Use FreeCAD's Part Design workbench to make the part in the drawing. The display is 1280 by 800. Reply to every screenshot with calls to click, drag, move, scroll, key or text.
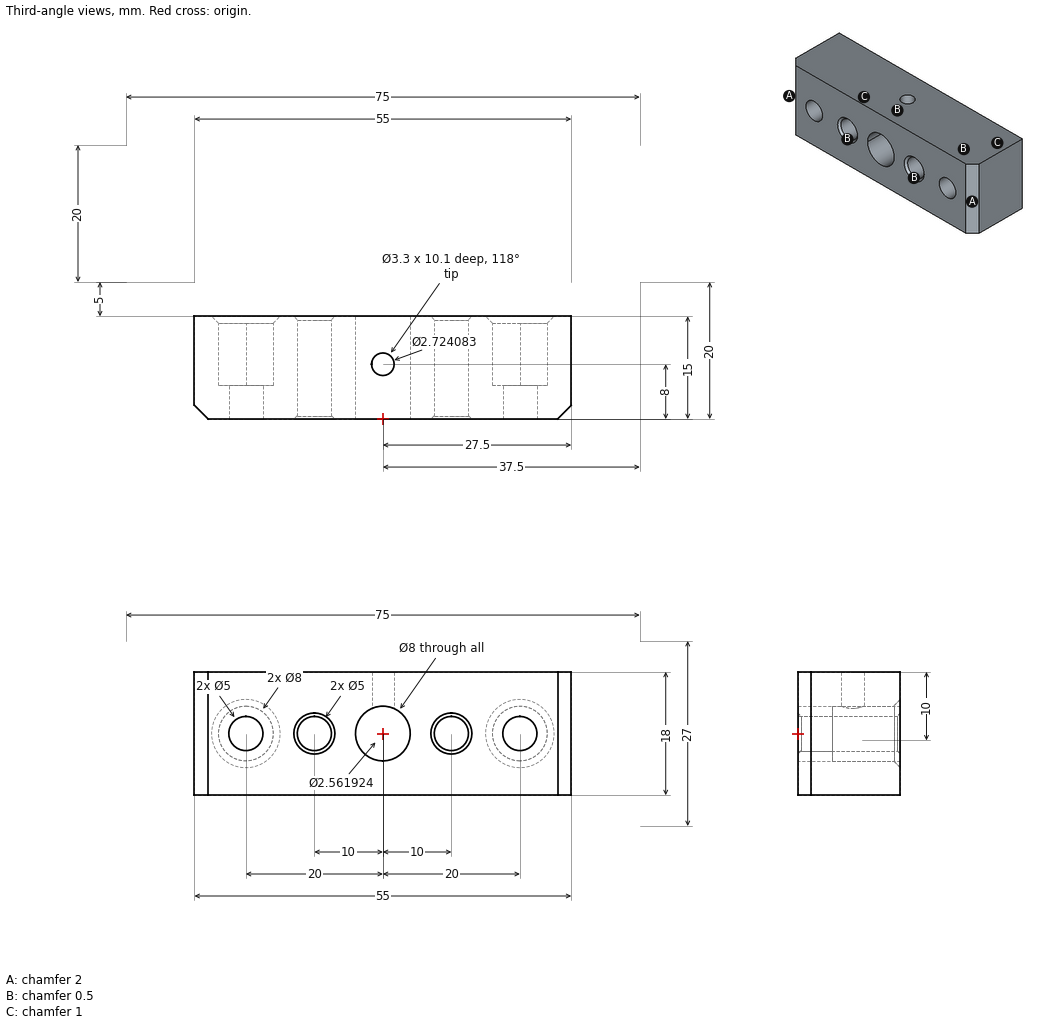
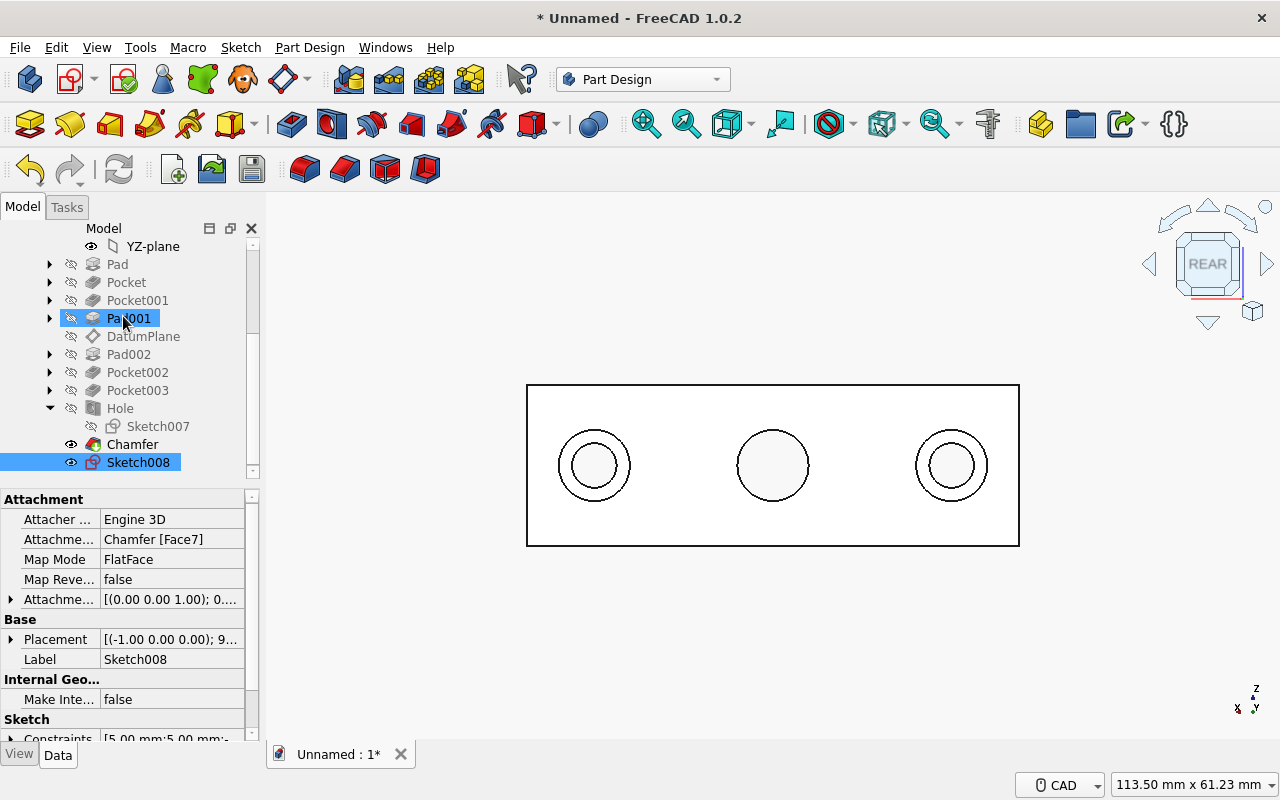
click(292, 124)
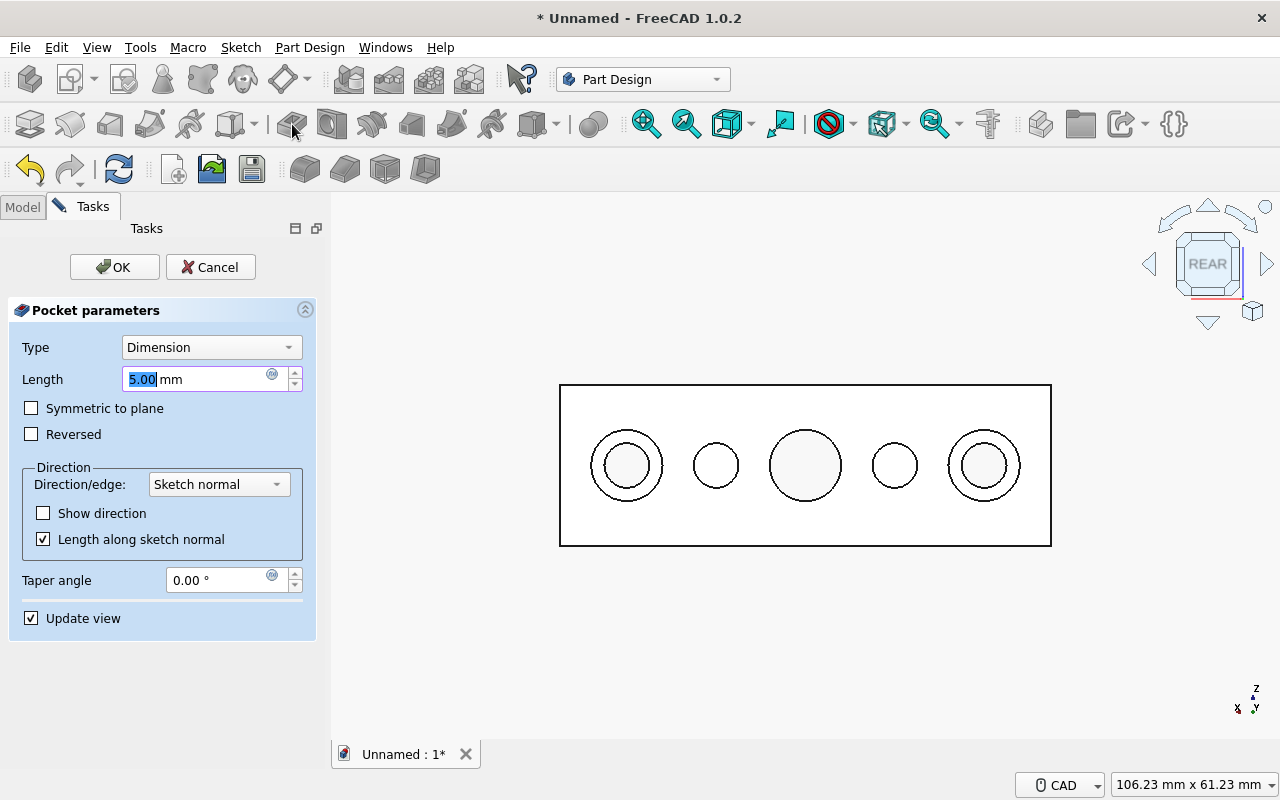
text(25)
key(Tab)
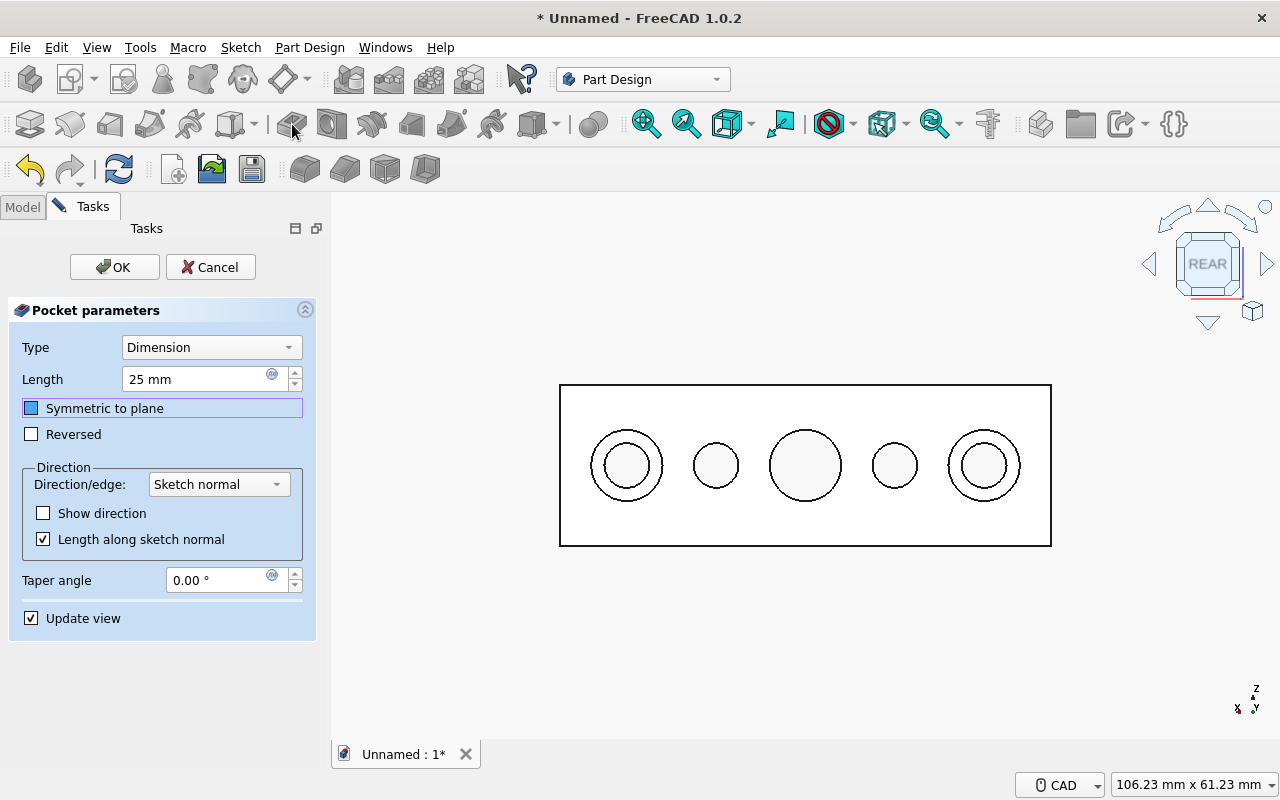
click(115, 267)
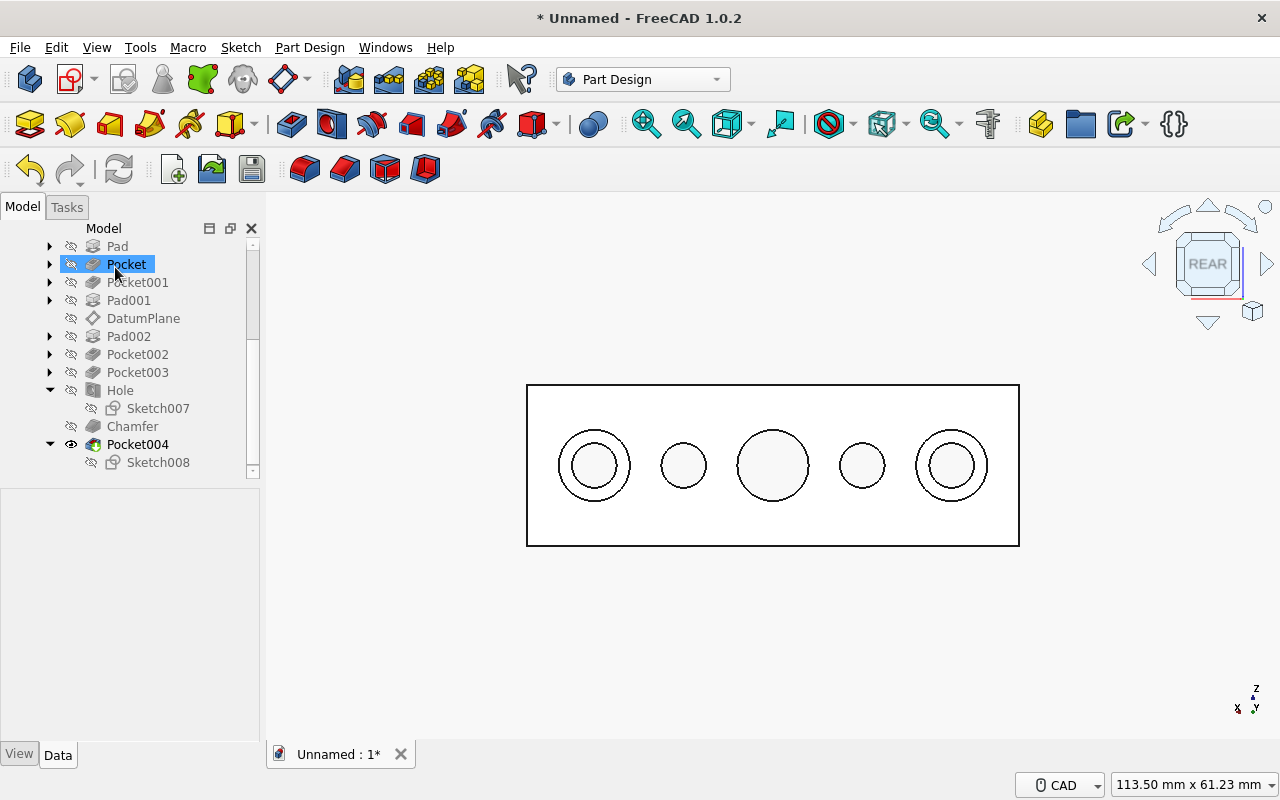
key(0)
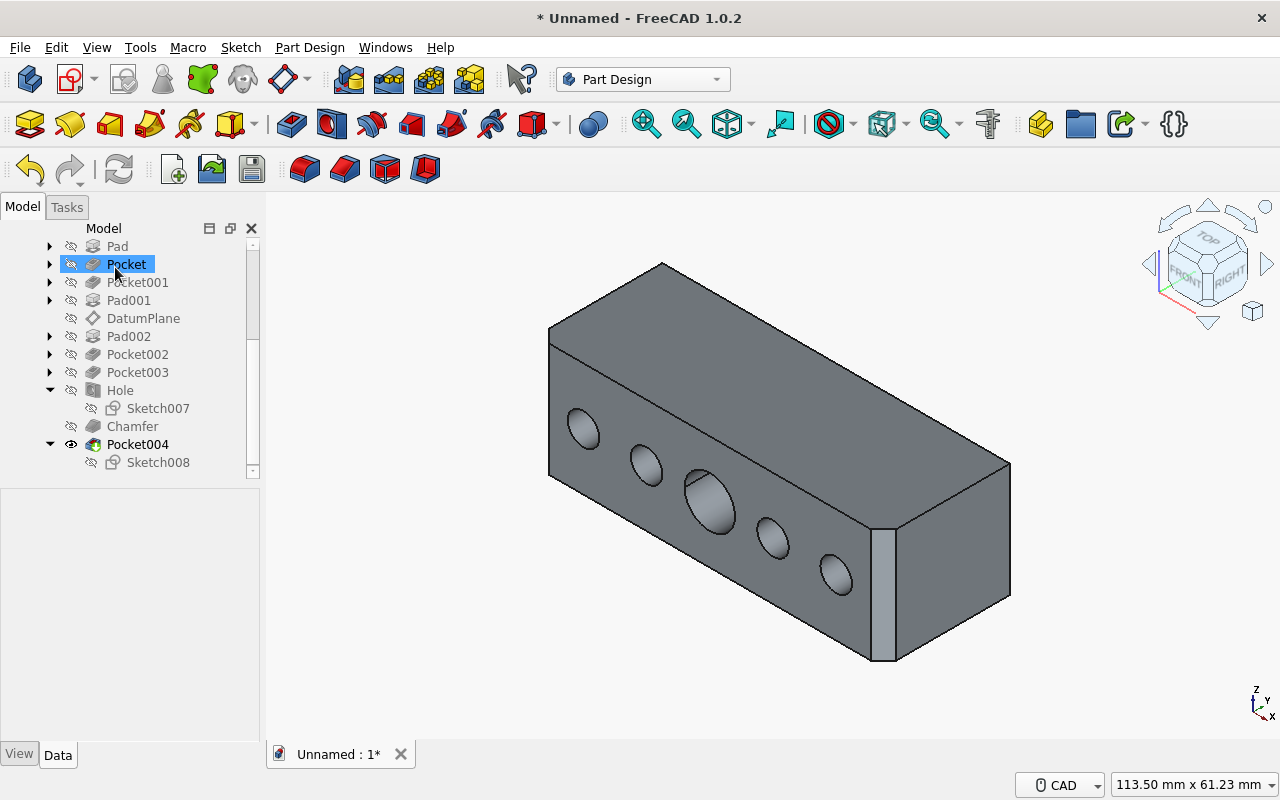
click(872, 456)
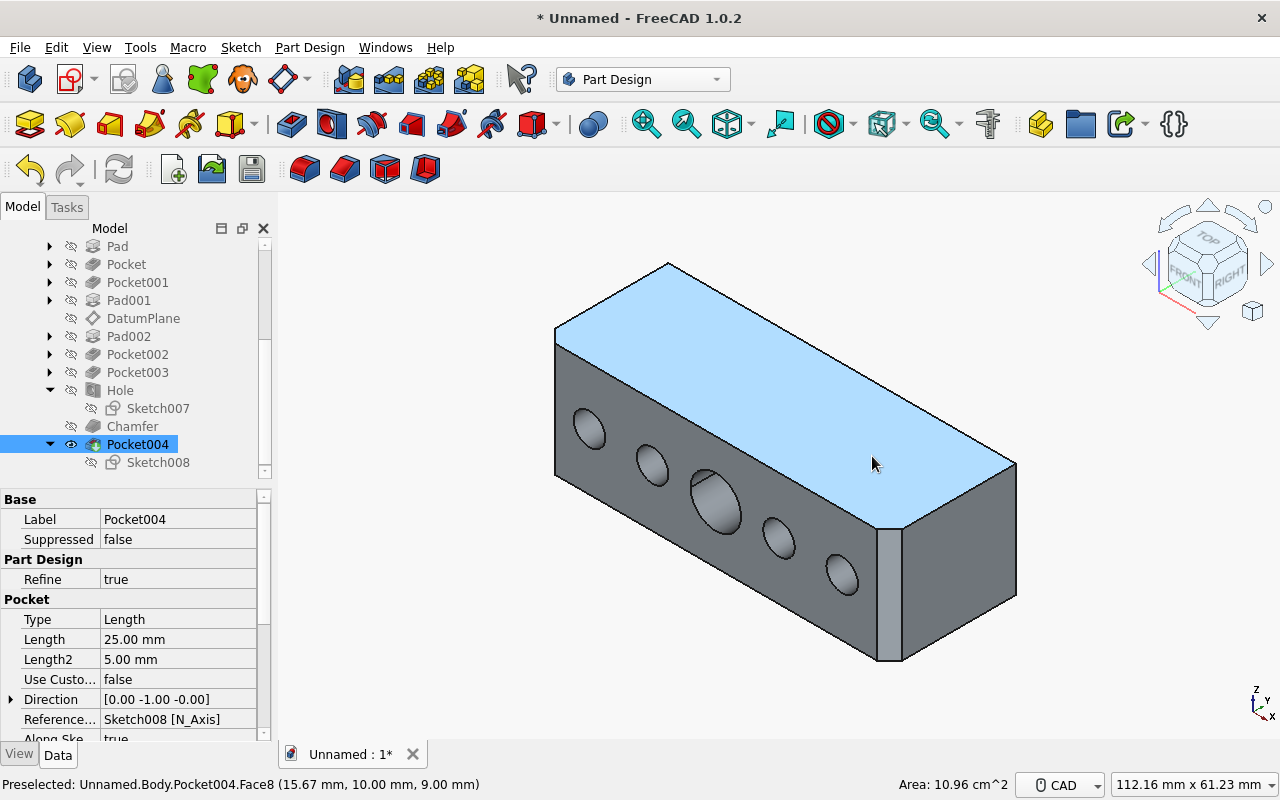
click(70, 80)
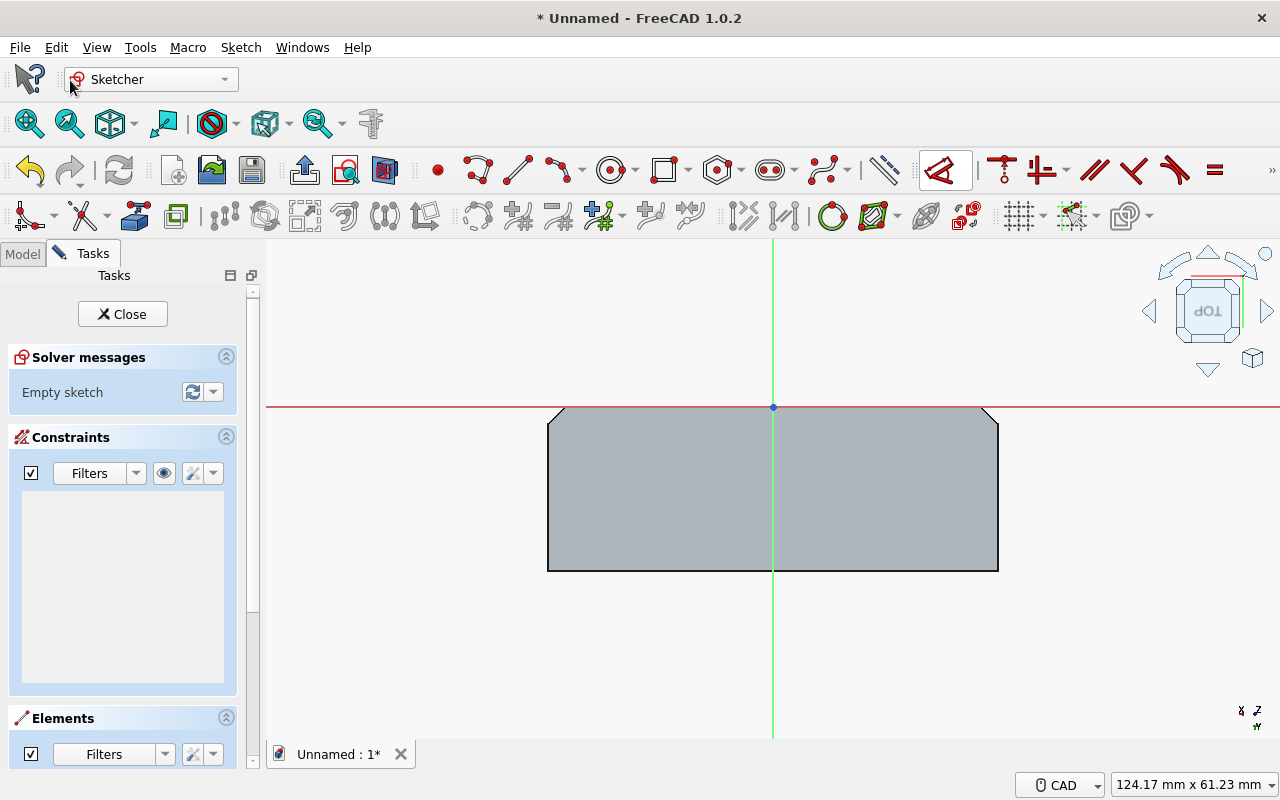
scroll(778, 471, up, 13)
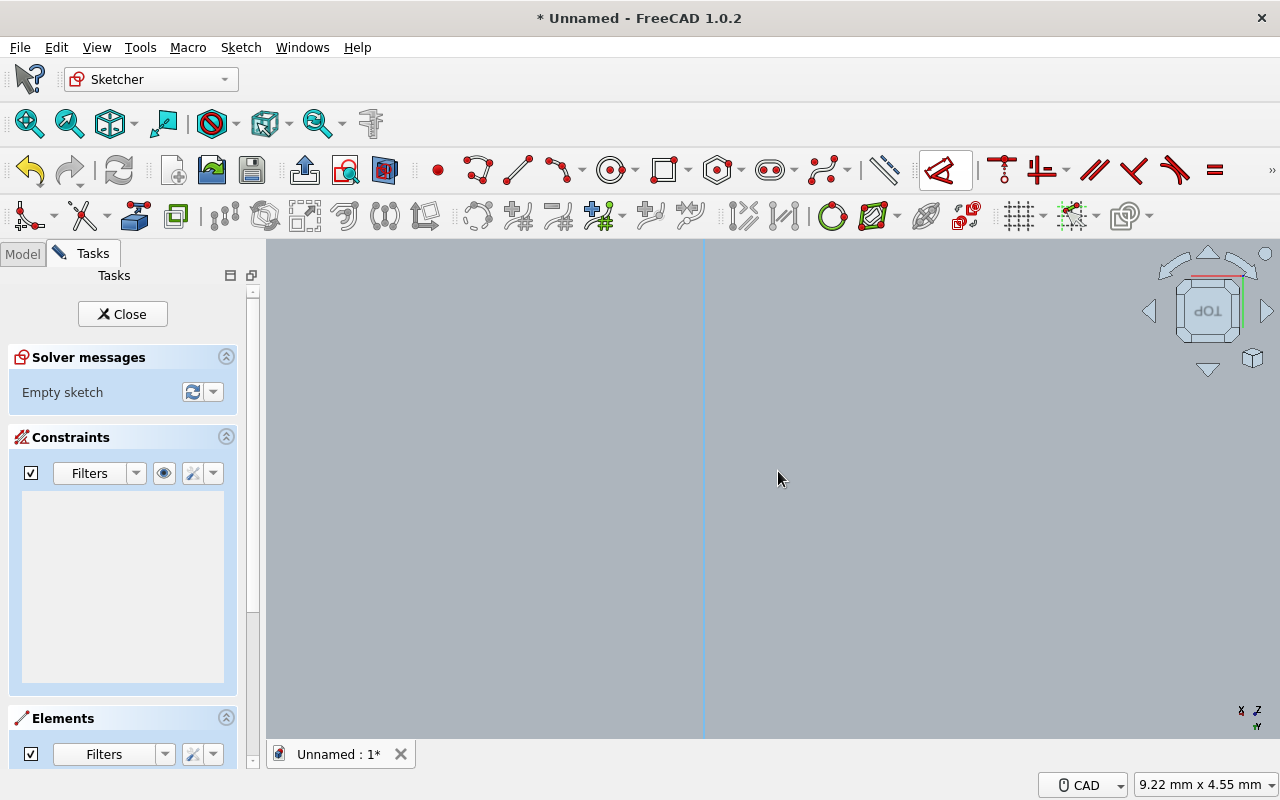
click(612, 170)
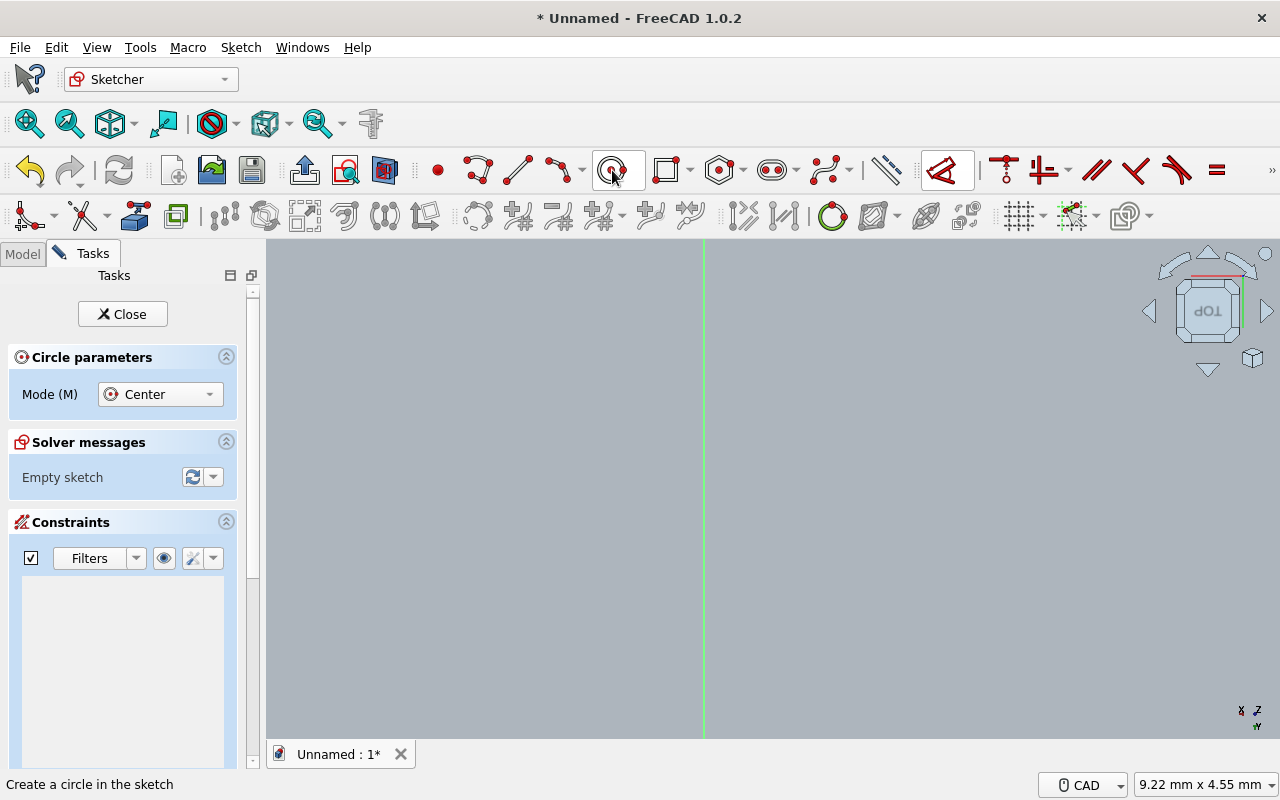
click(704, 488)
move(810, 382)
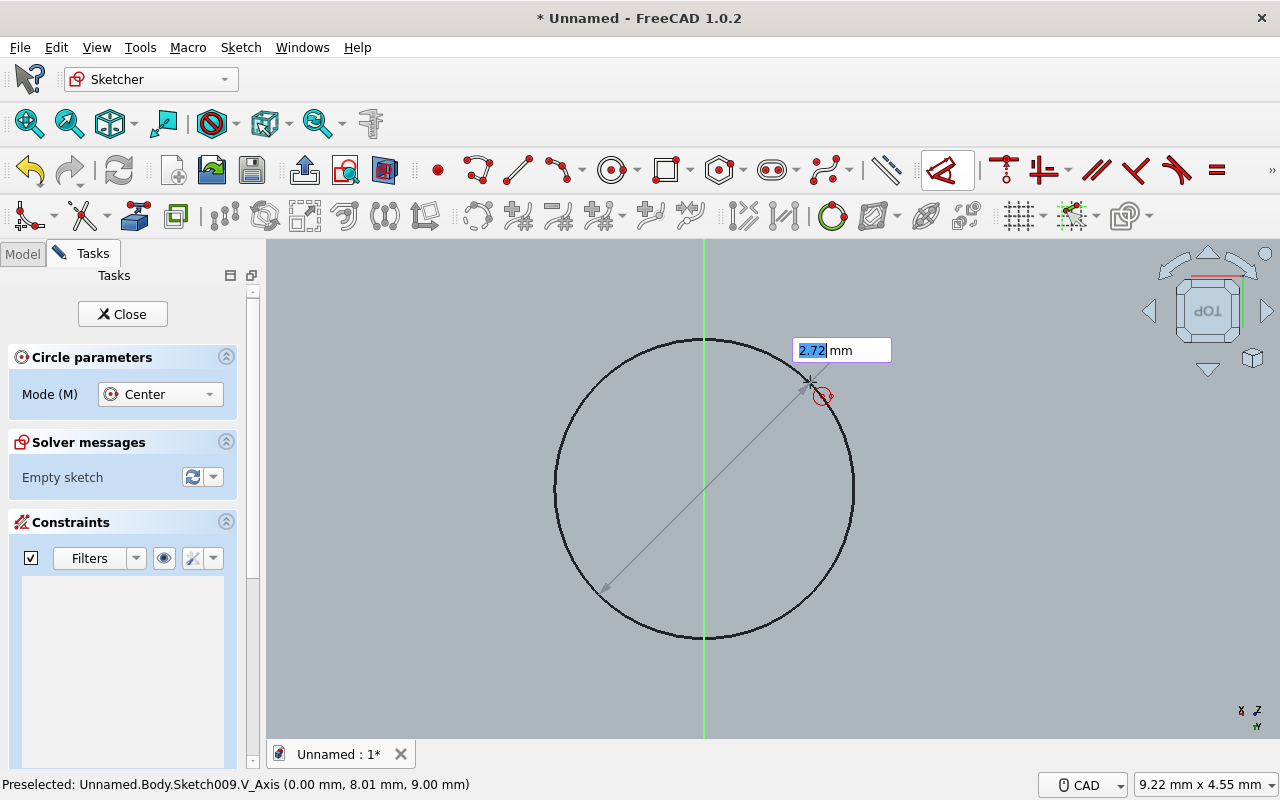
text(2.724083)
key(Return)
key(Escape)